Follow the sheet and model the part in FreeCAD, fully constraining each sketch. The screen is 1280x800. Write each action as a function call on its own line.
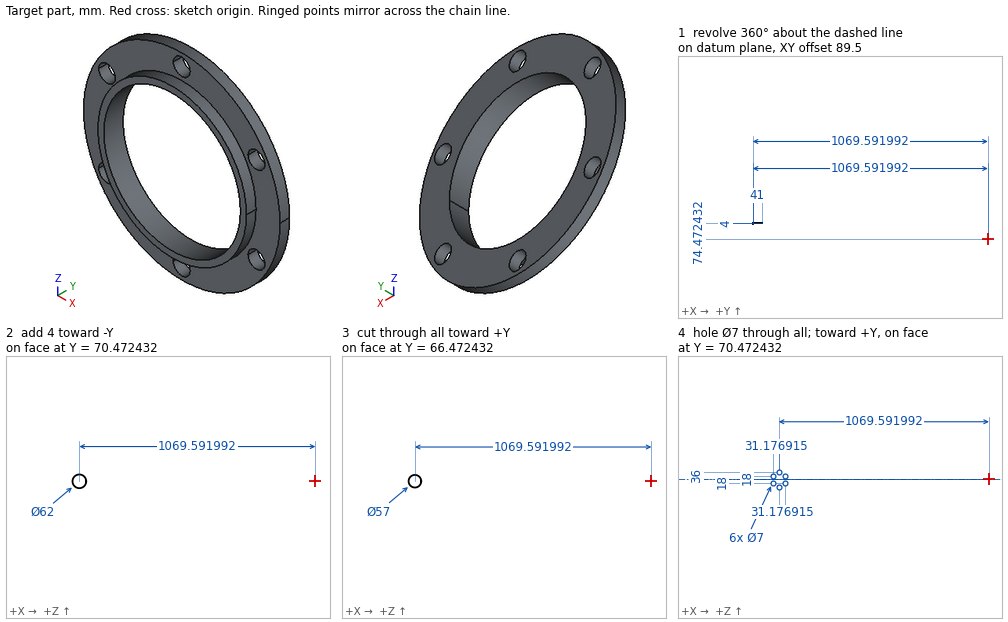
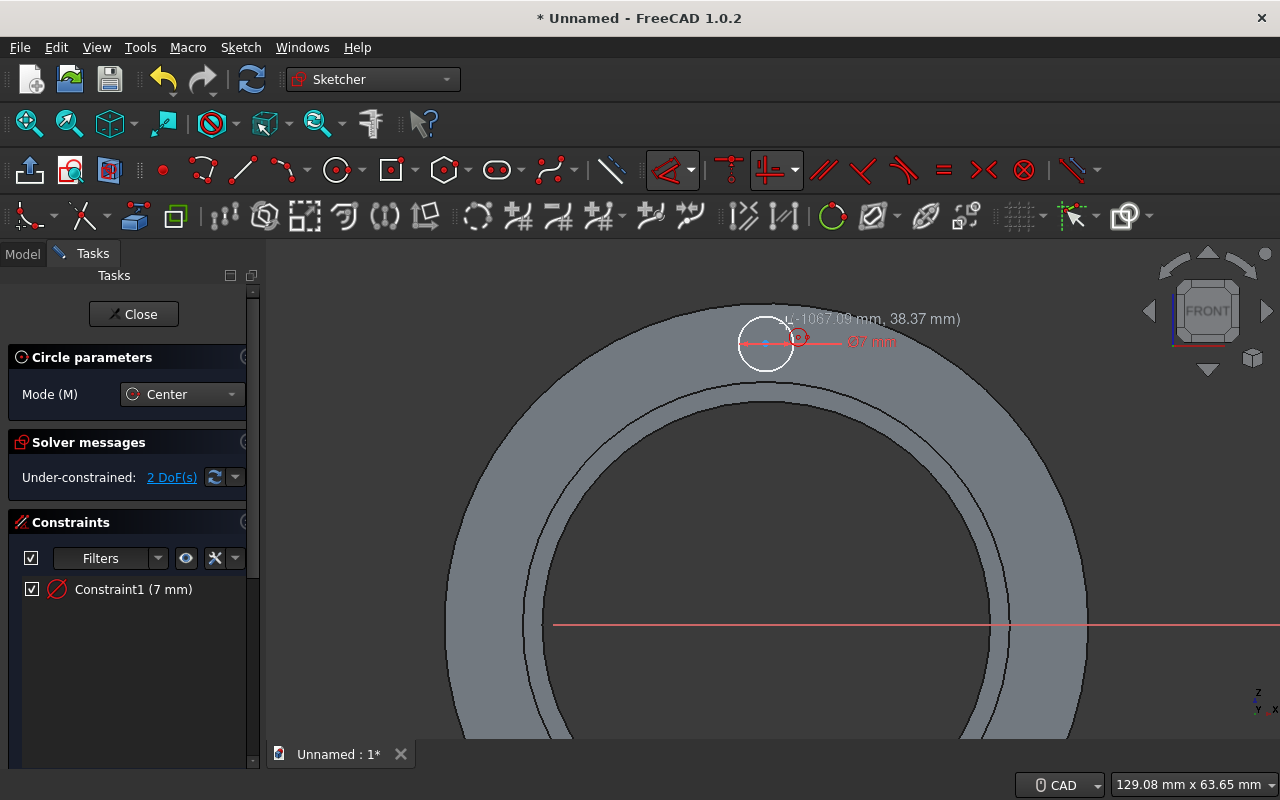
click(521, 484)
move(541, 465)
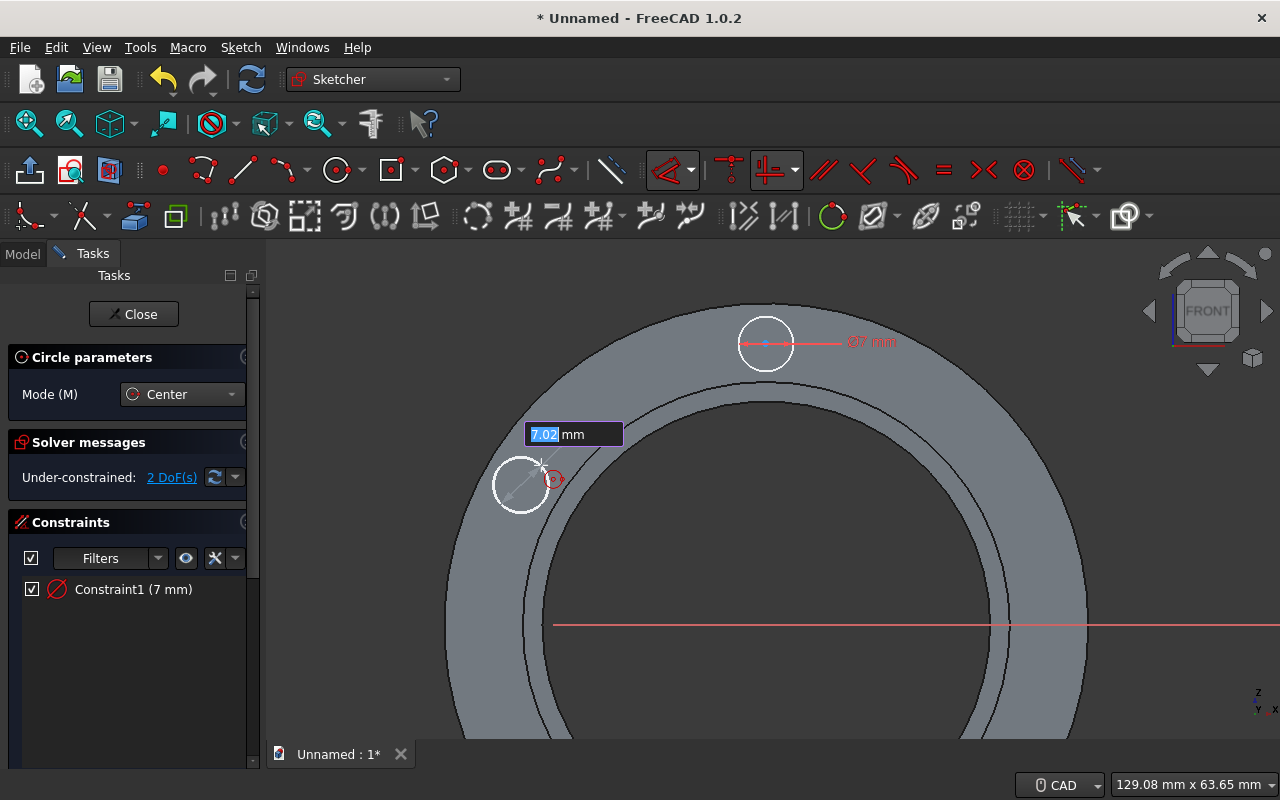
text(7)
key(Return)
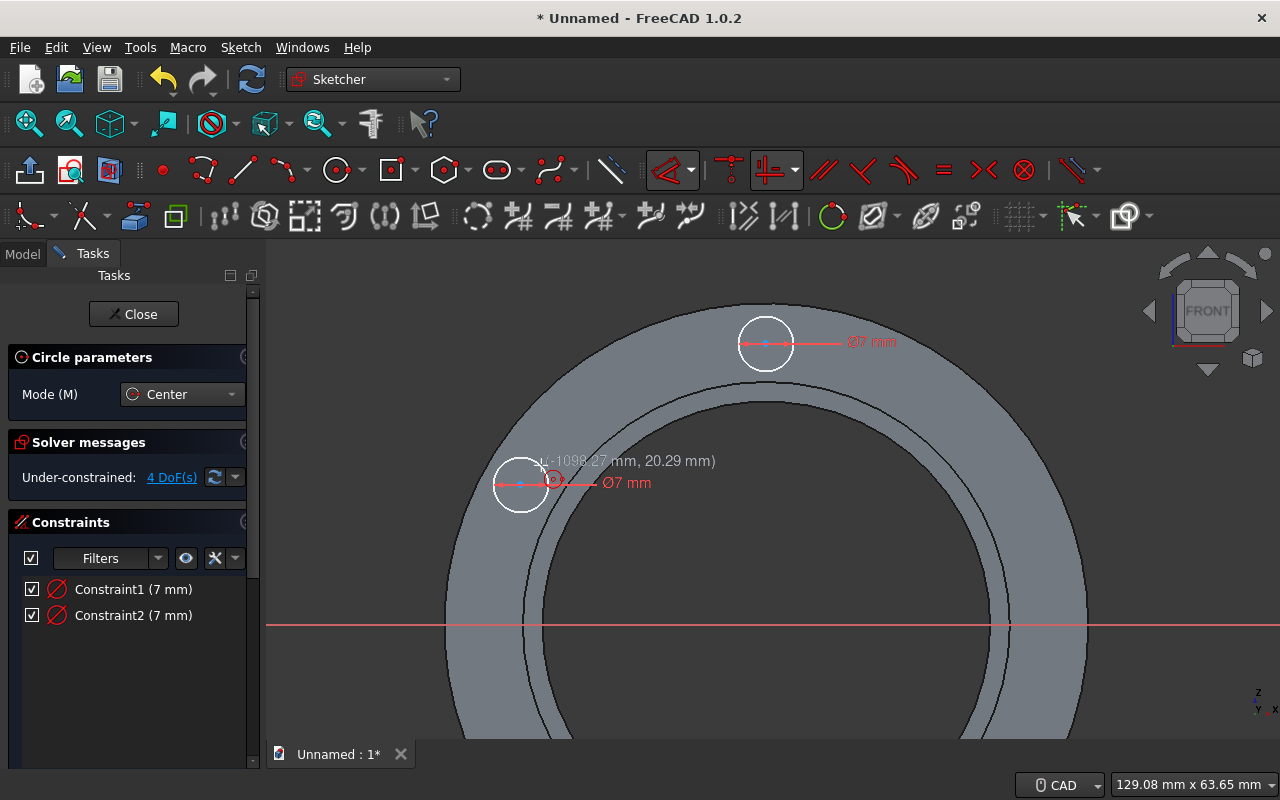
scroll(629, 323, down, 3)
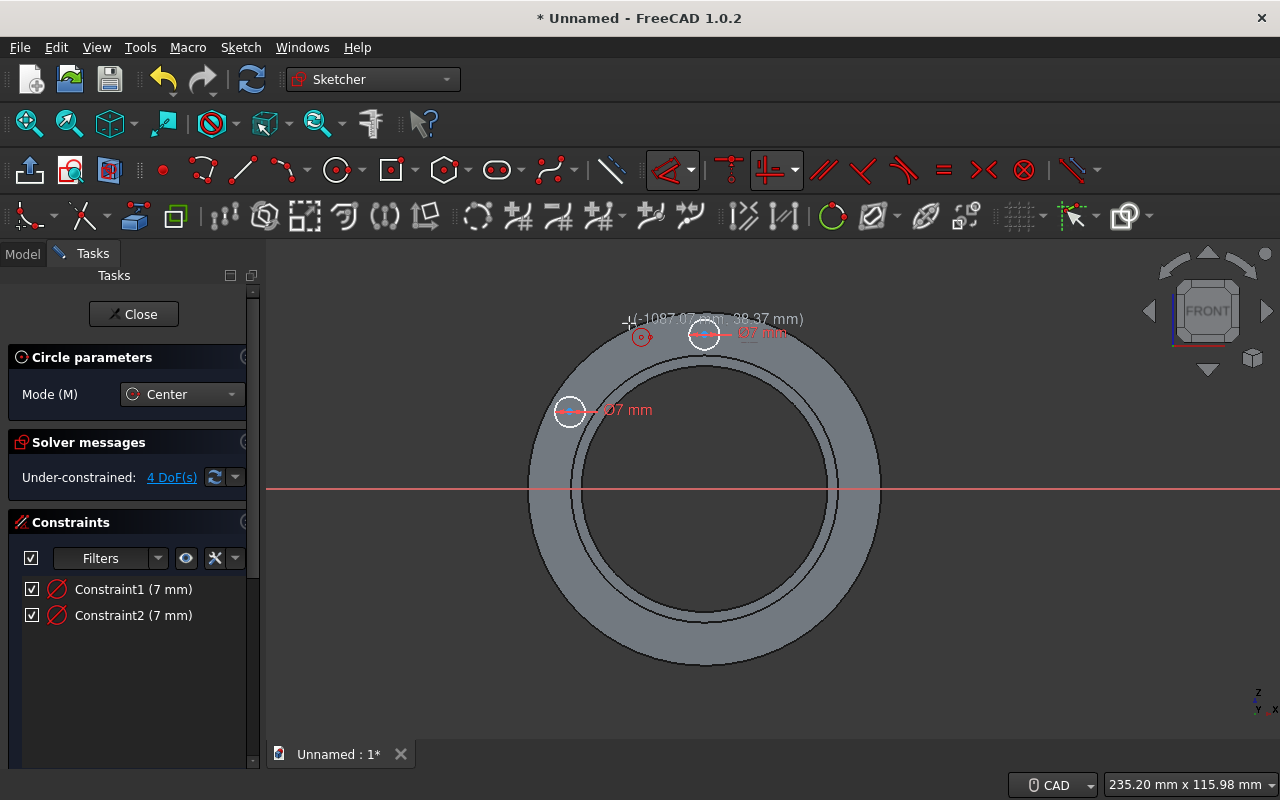
scroll(570, 567, up, 3)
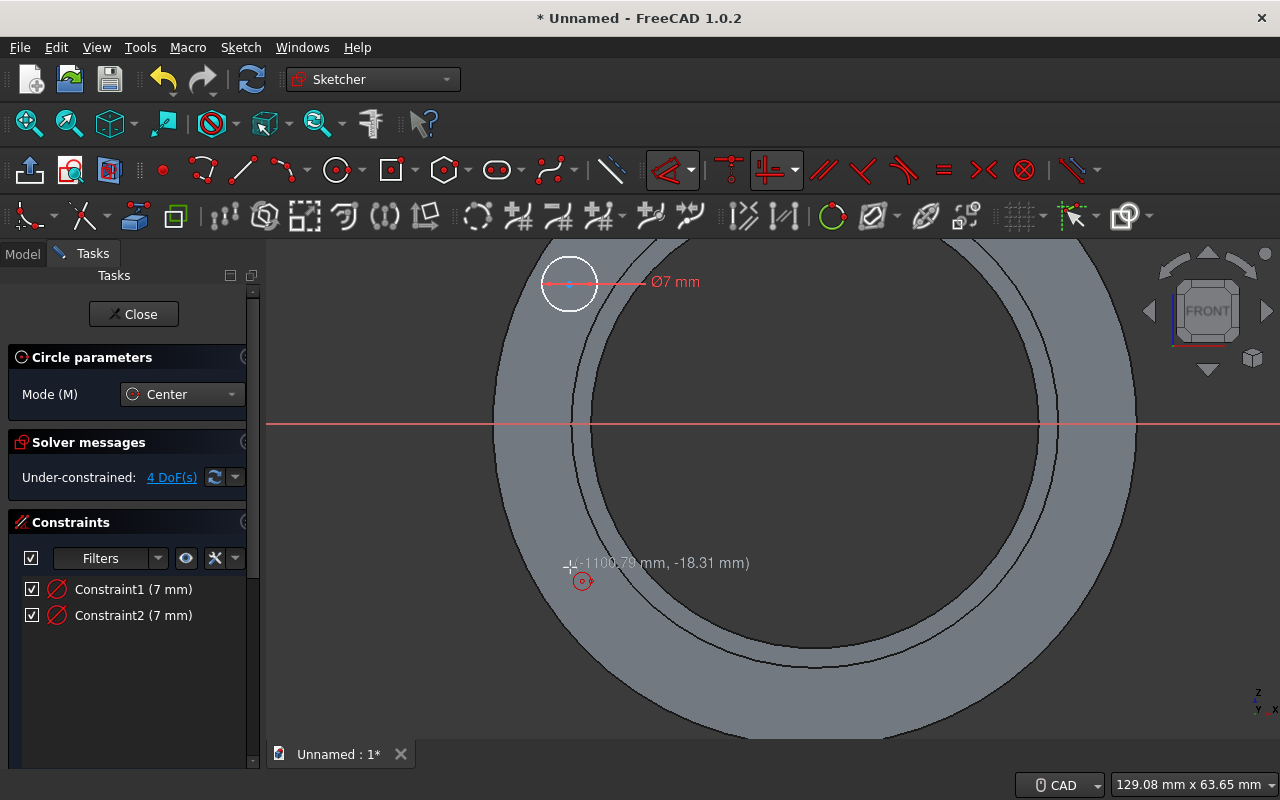
click(570, 566)
move(589, 546)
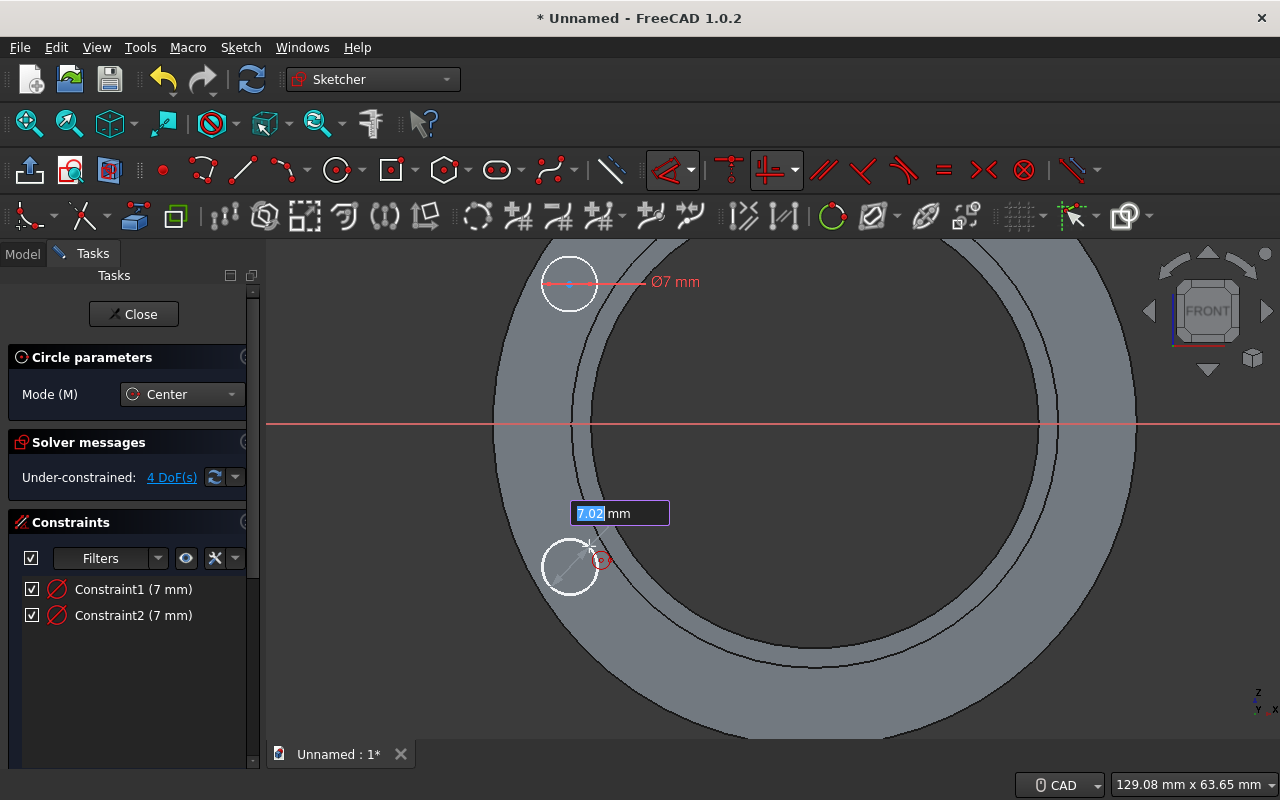
text(7)
key(Return)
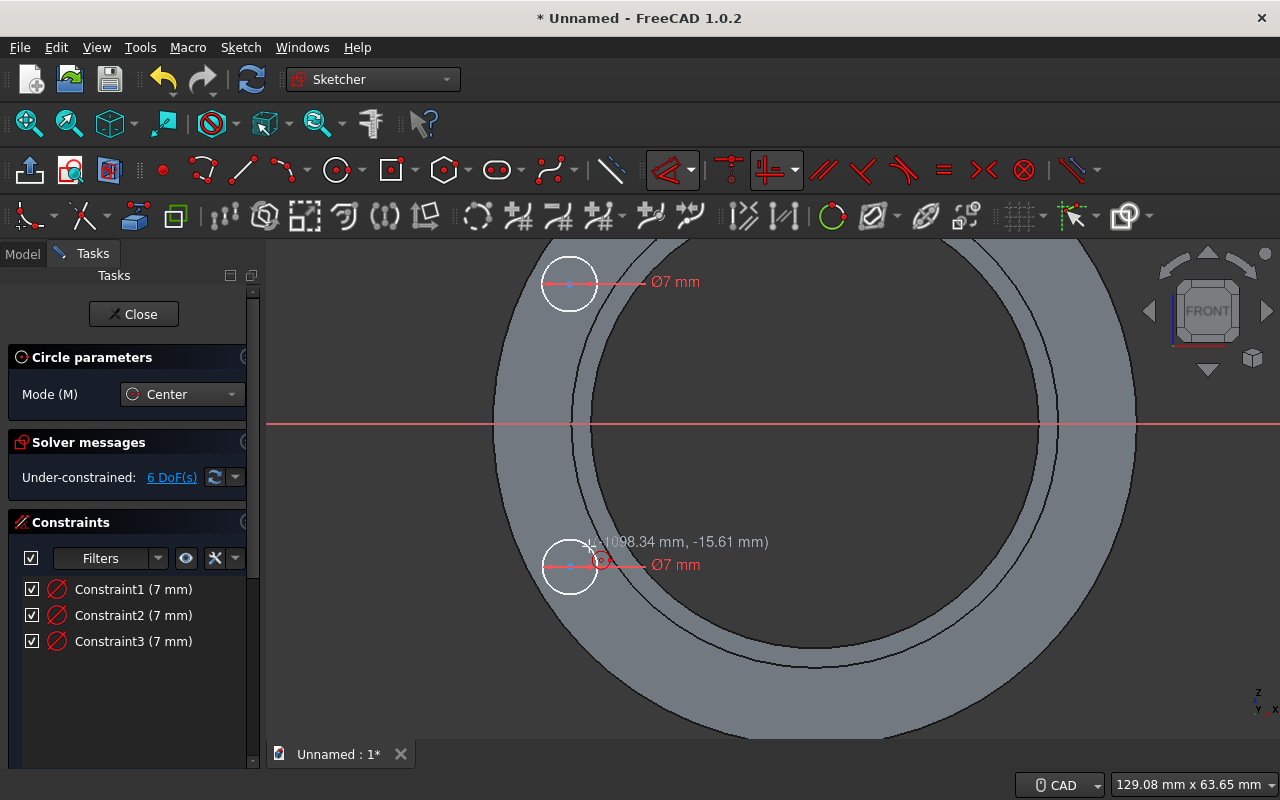
click(815, 707)
move(834, 688)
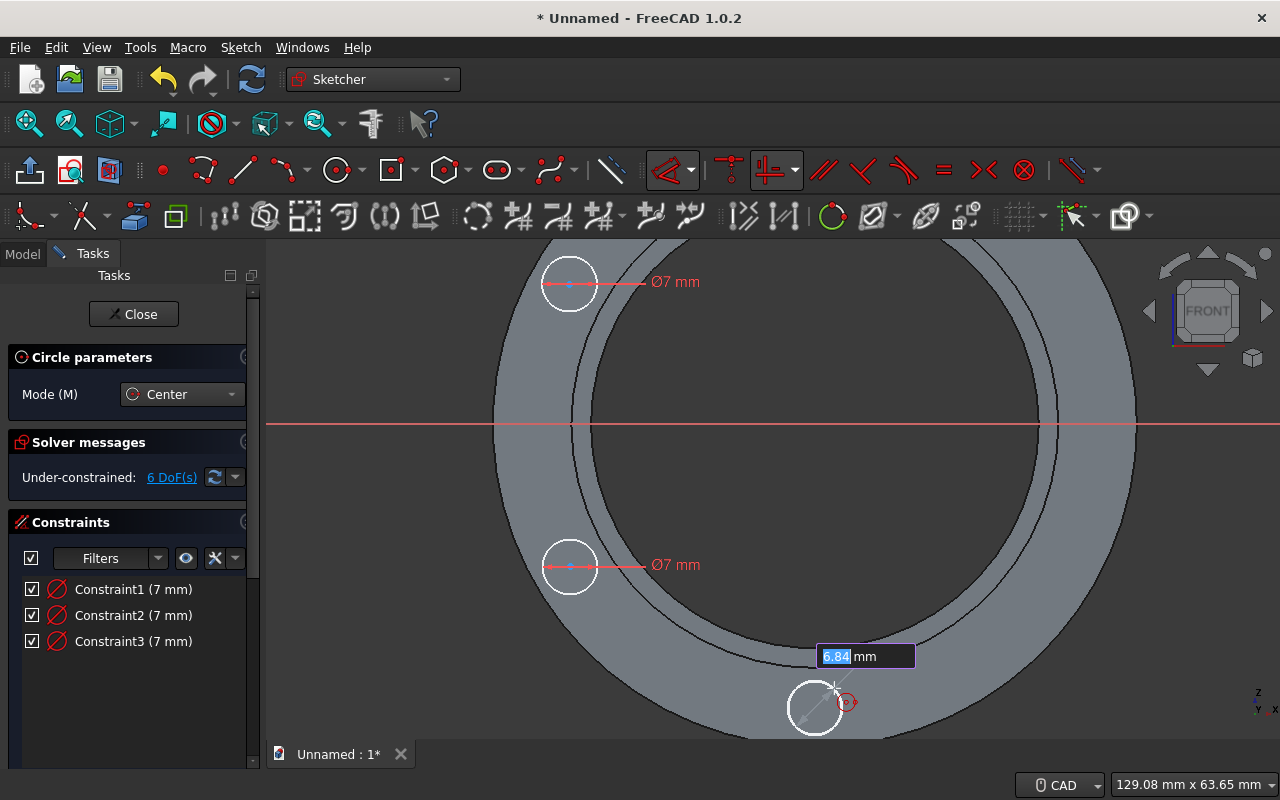
text(7)
key(Return)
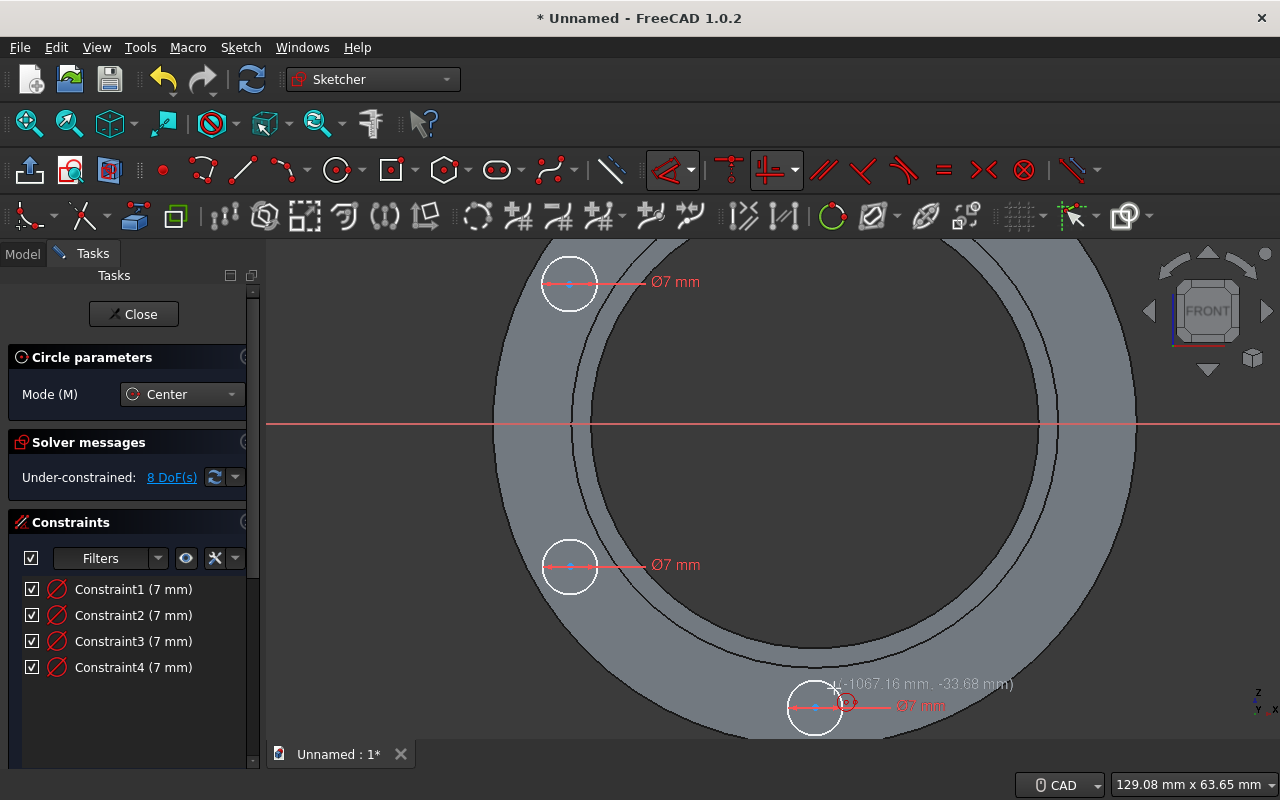
click(1060, 566)
move(1079, 546)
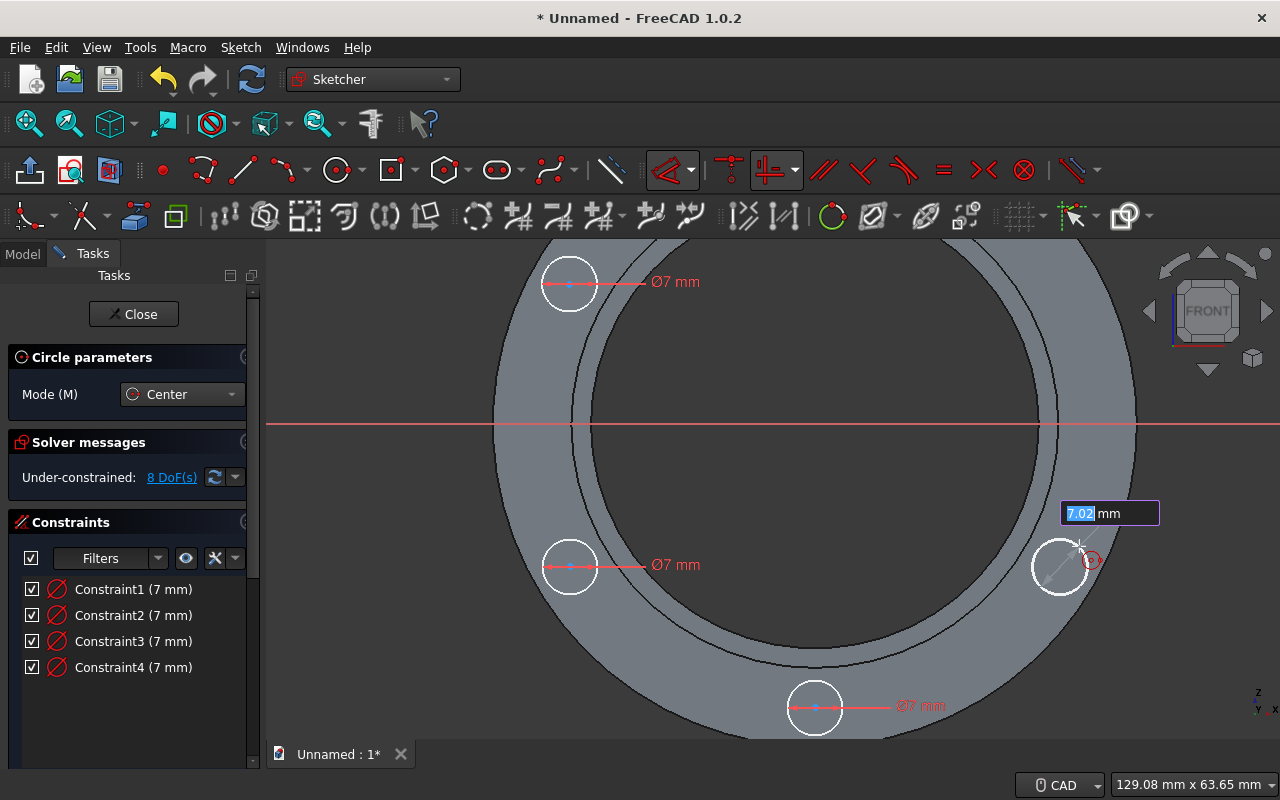
text(7)
key(Return)